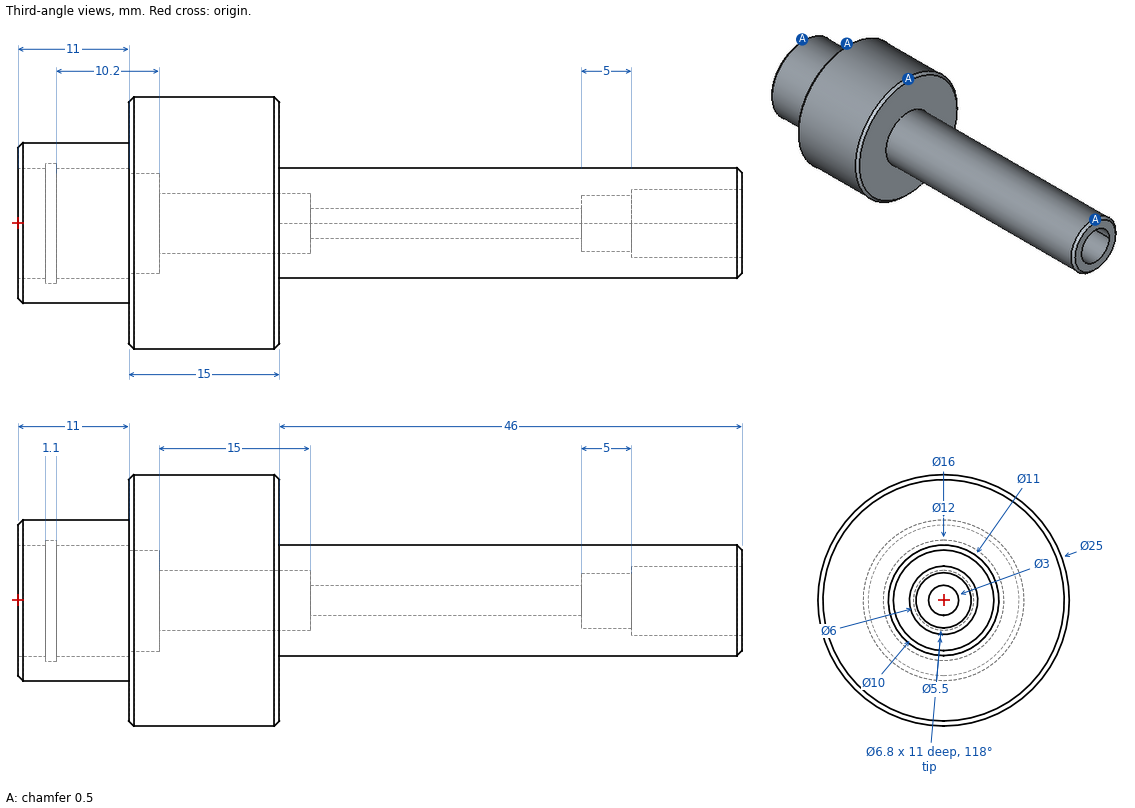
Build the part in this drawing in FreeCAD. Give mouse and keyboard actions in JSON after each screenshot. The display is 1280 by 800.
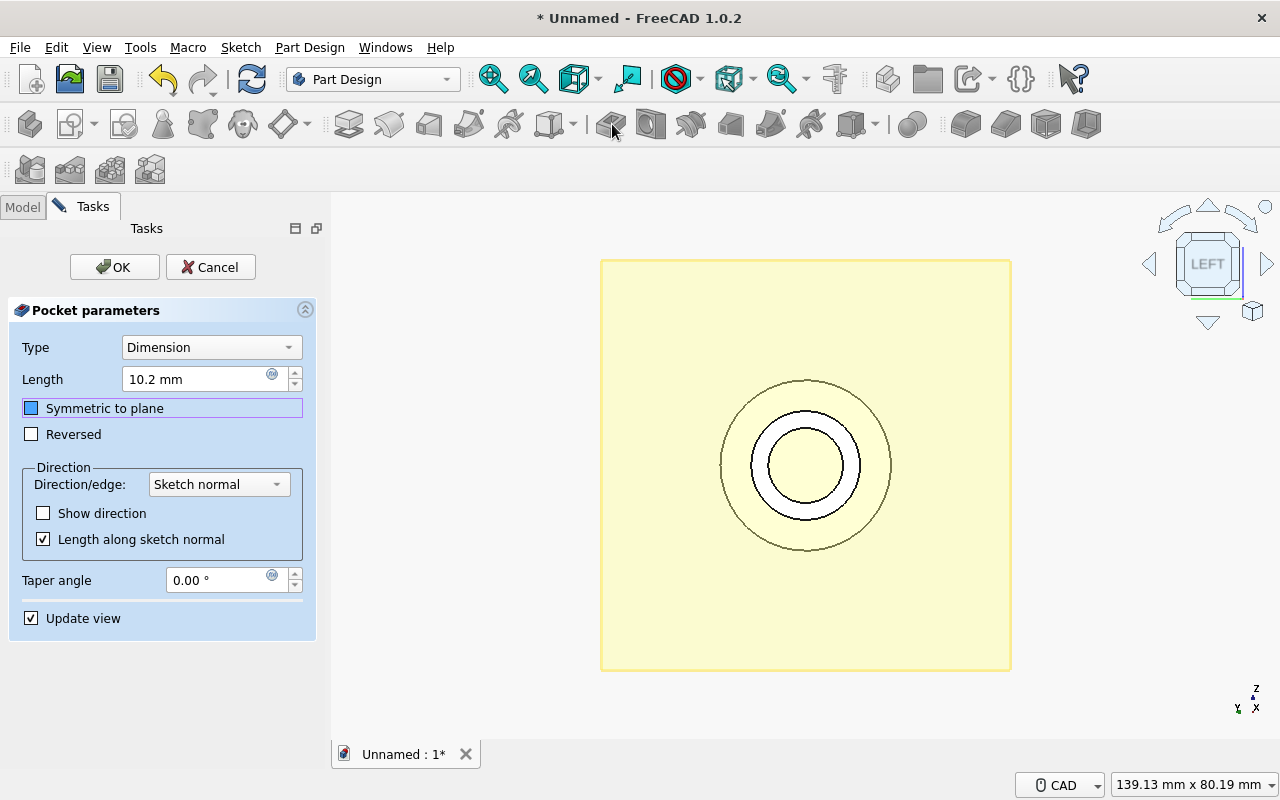
{"action": "left_click", "coordinate": [30, 434]}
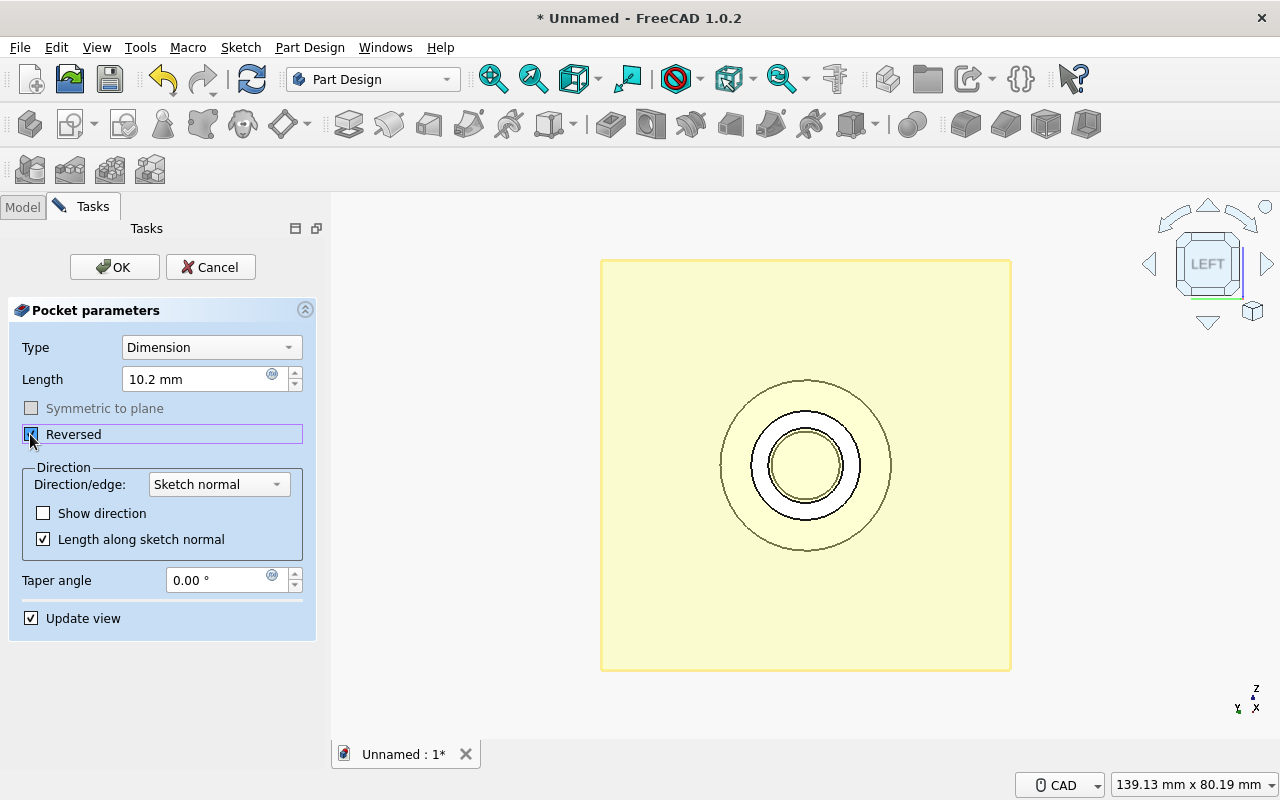
{"action": "left_click", "coordinate": [115, 267]}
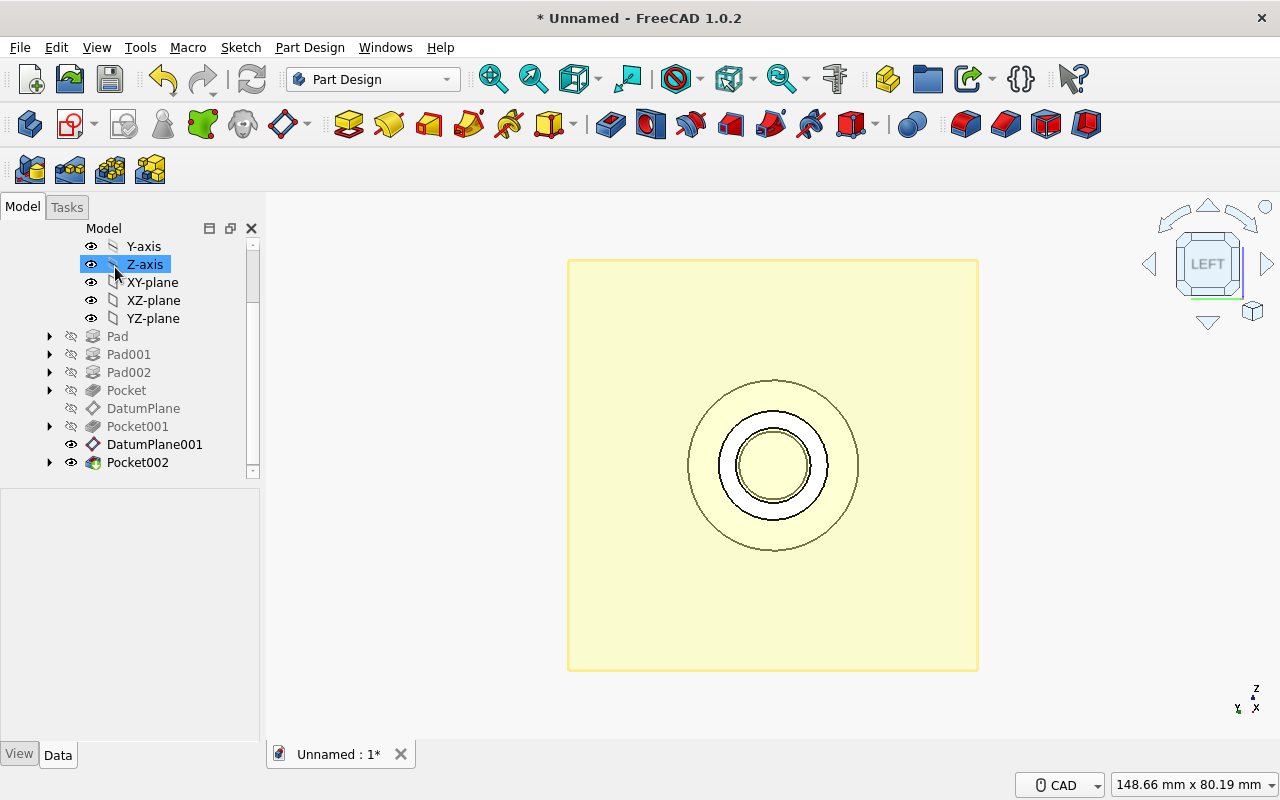
{"action": "left_click", "coordinate": [116, 444]}
{"action": "key", "text": "space"}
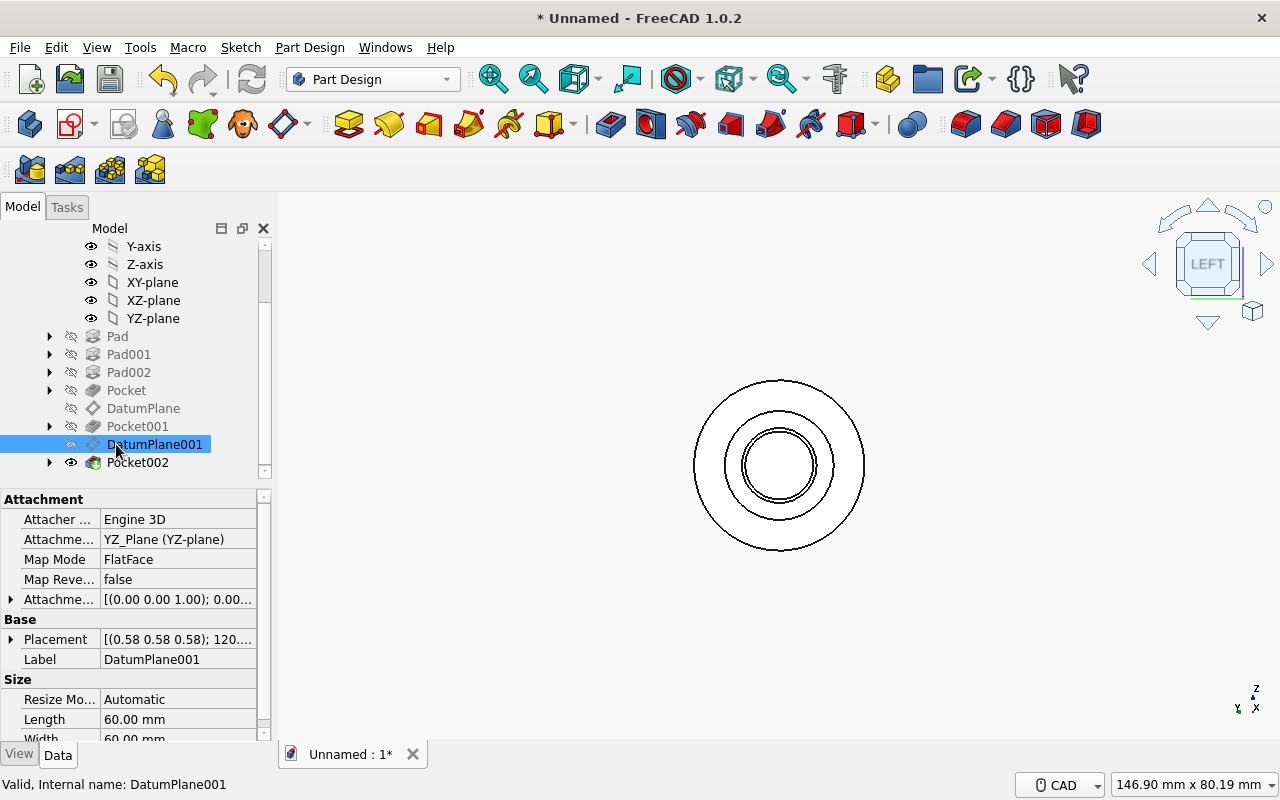
{"action": "left_click", "coordinate": [494, 80]}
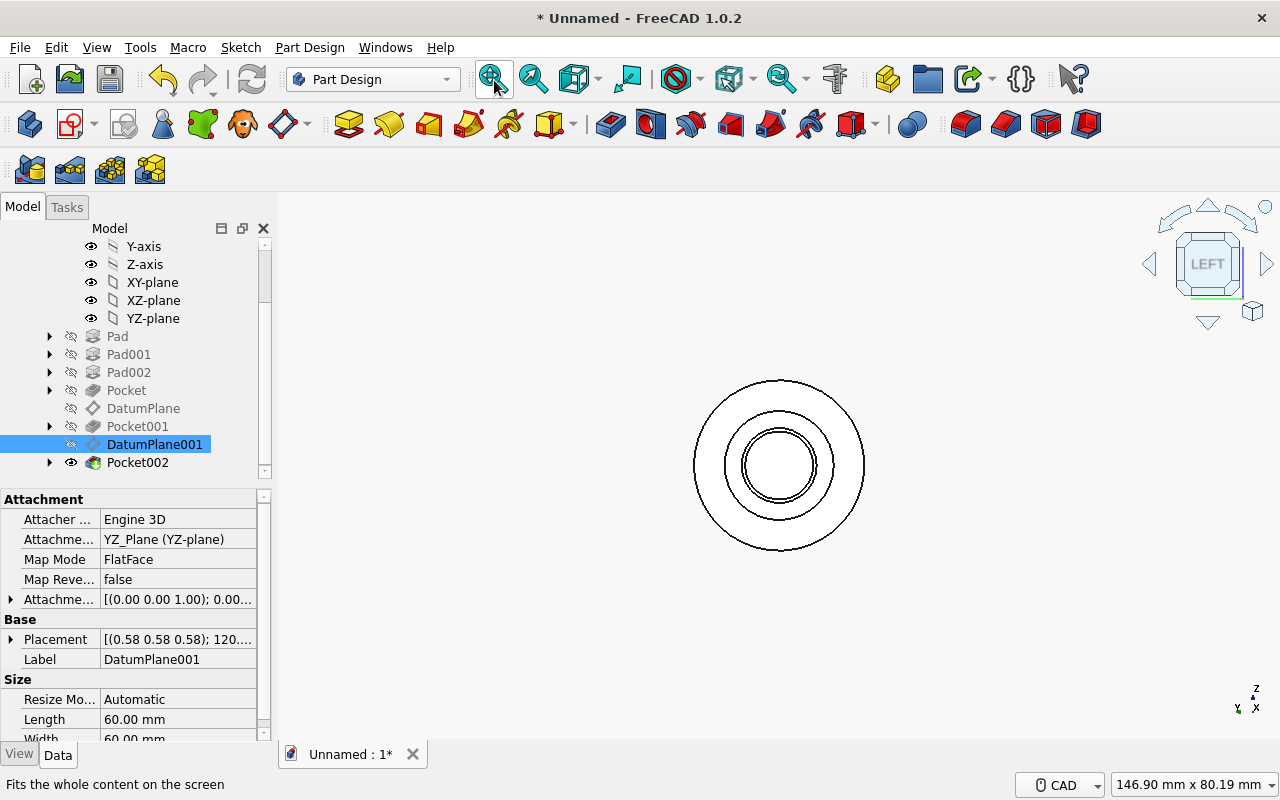
{"action": "left_click", "coordinate": [779, 464]}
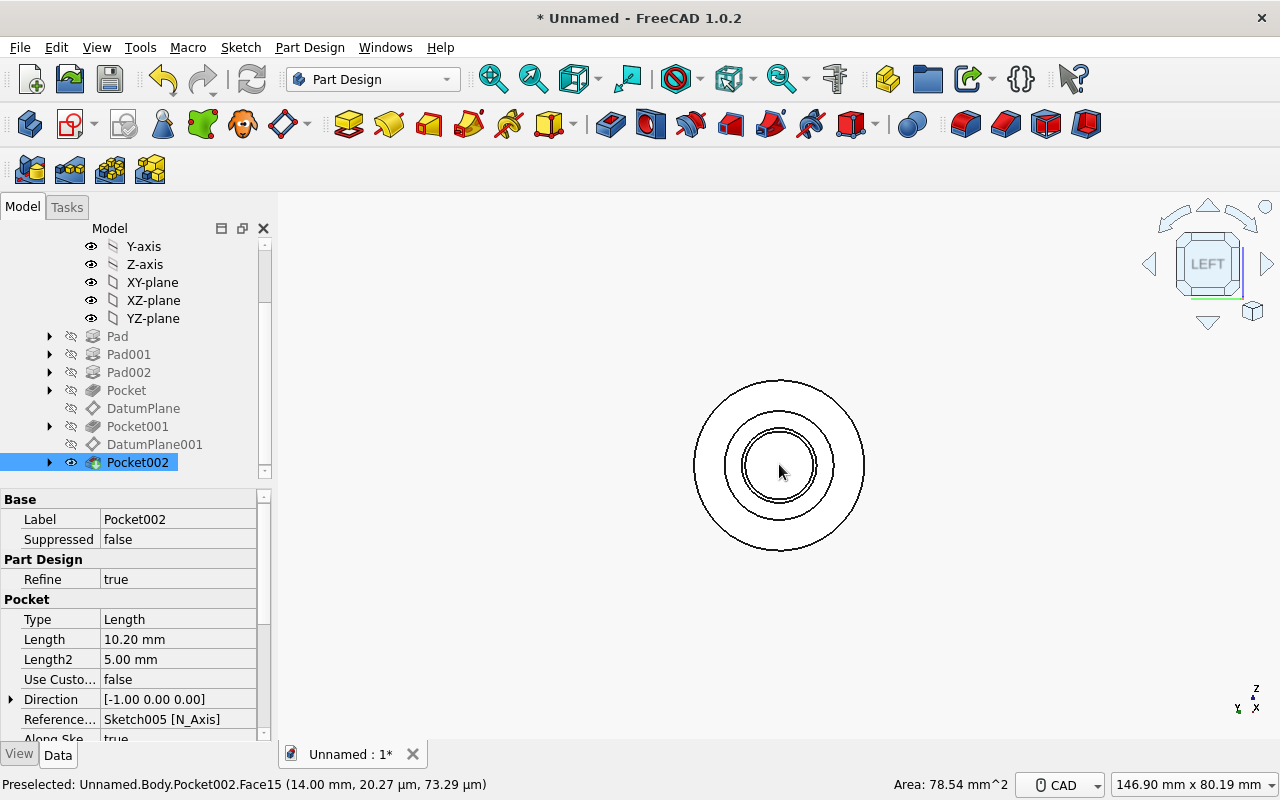
{"action": "left_click", "coordinate": [70, 124]}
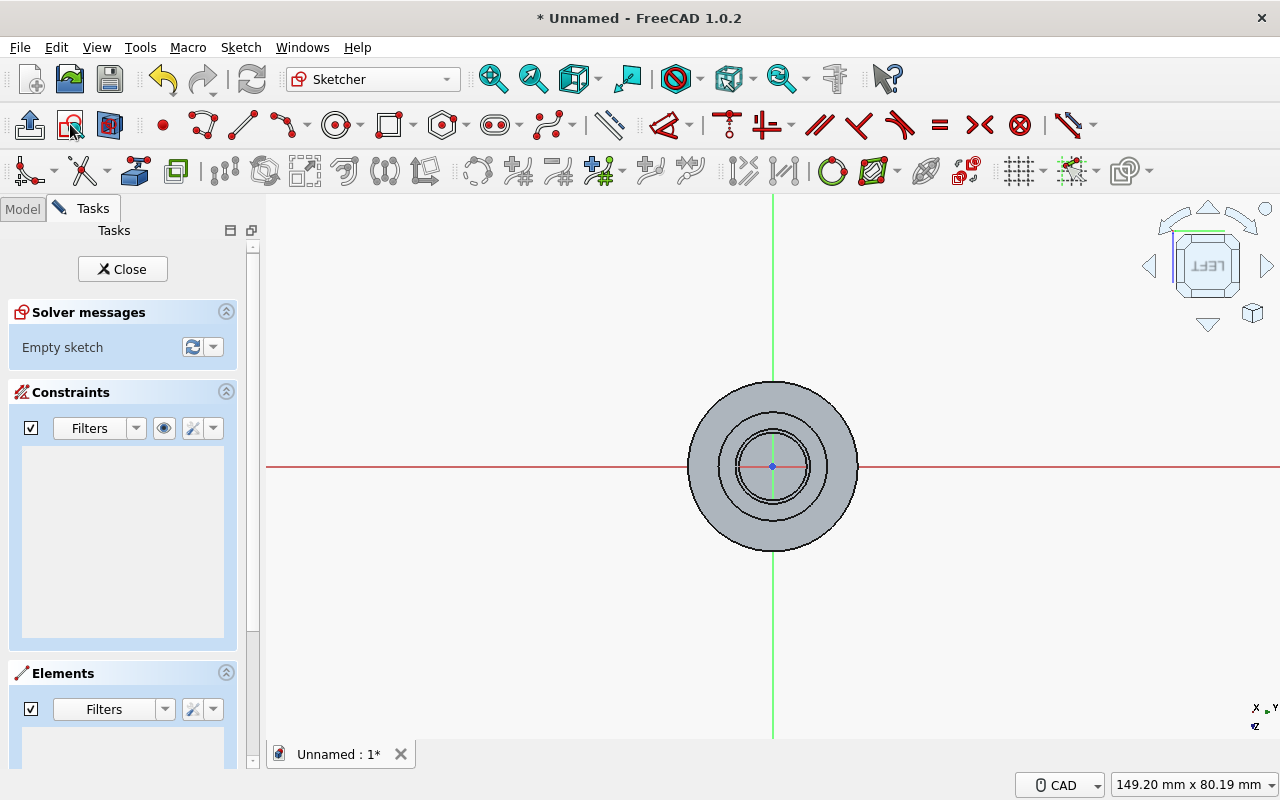
{"action": "left_click", "coordinate": [110, 126]}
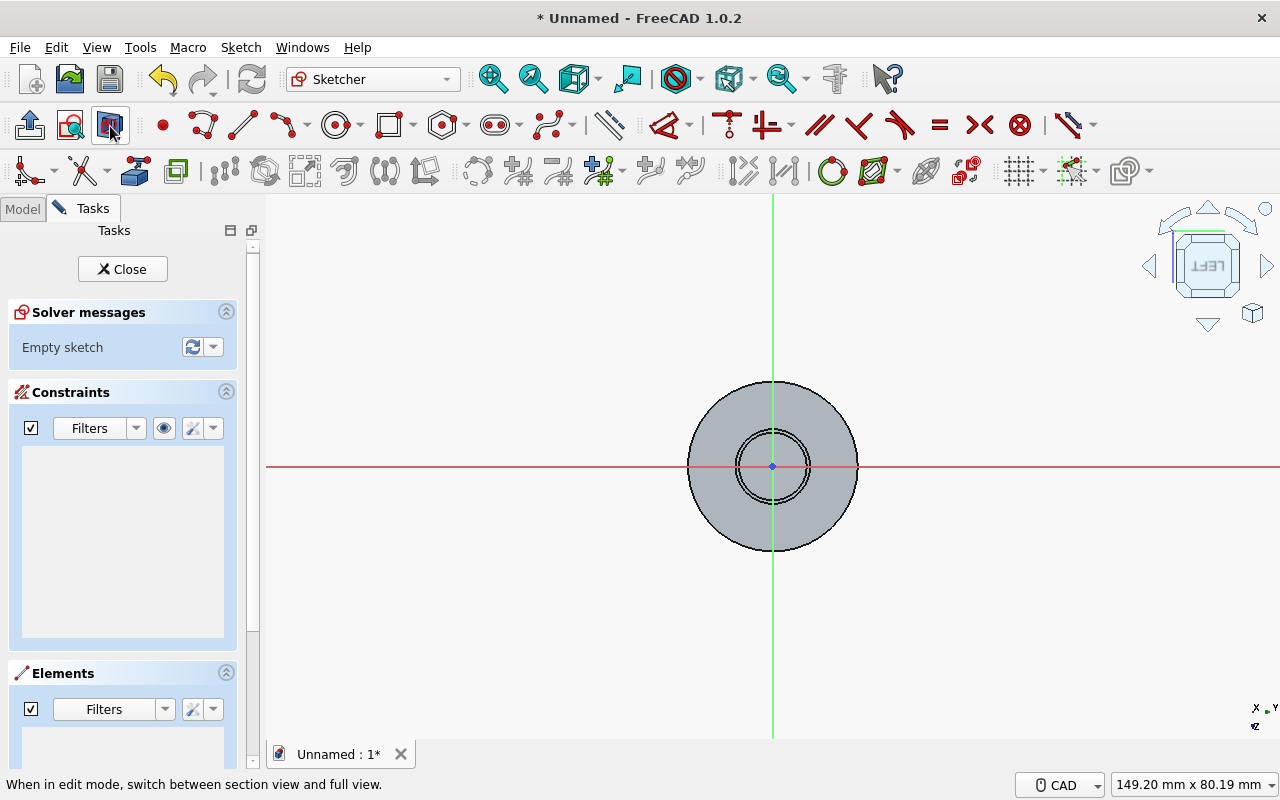
{"action": "scroll", "coordinate": [781, 466], "scroll_direction": "up", "scroll_amount": 11}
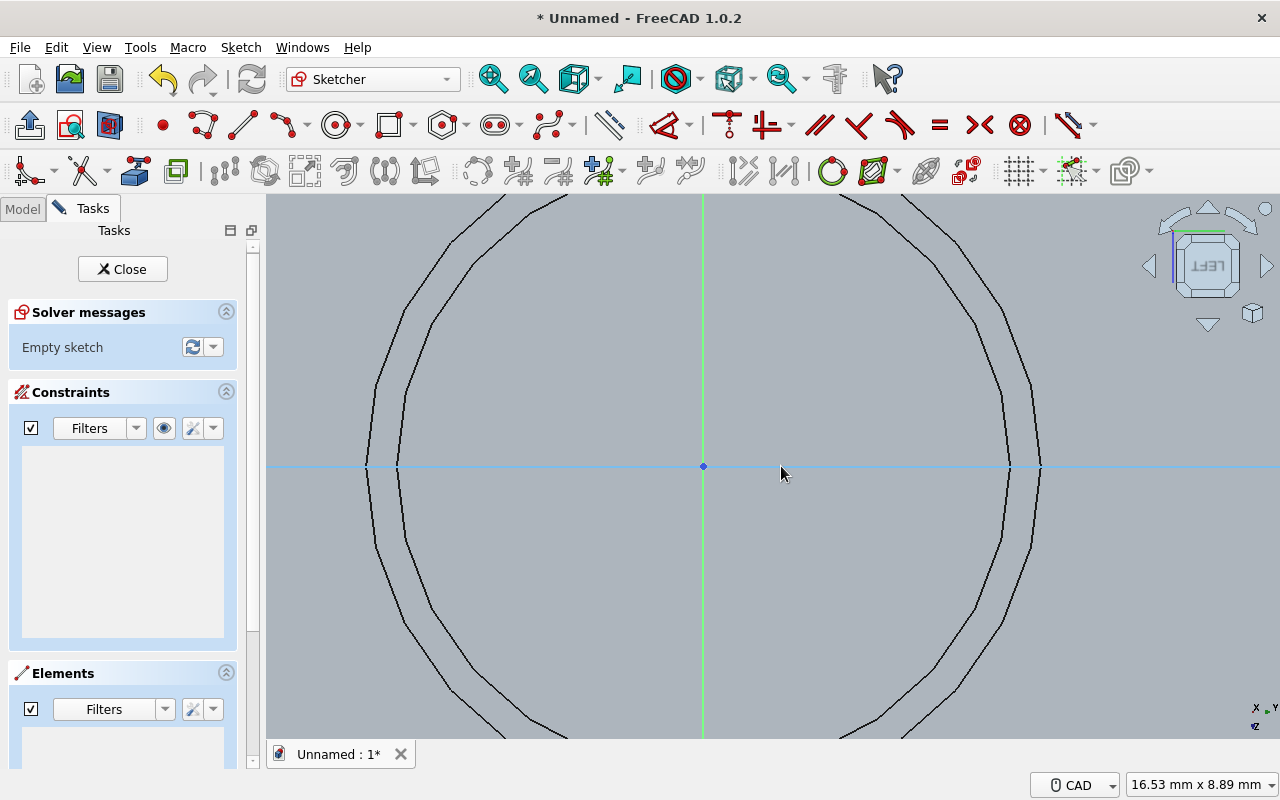
{"action": "left_click", "coordinate": [336, 126]}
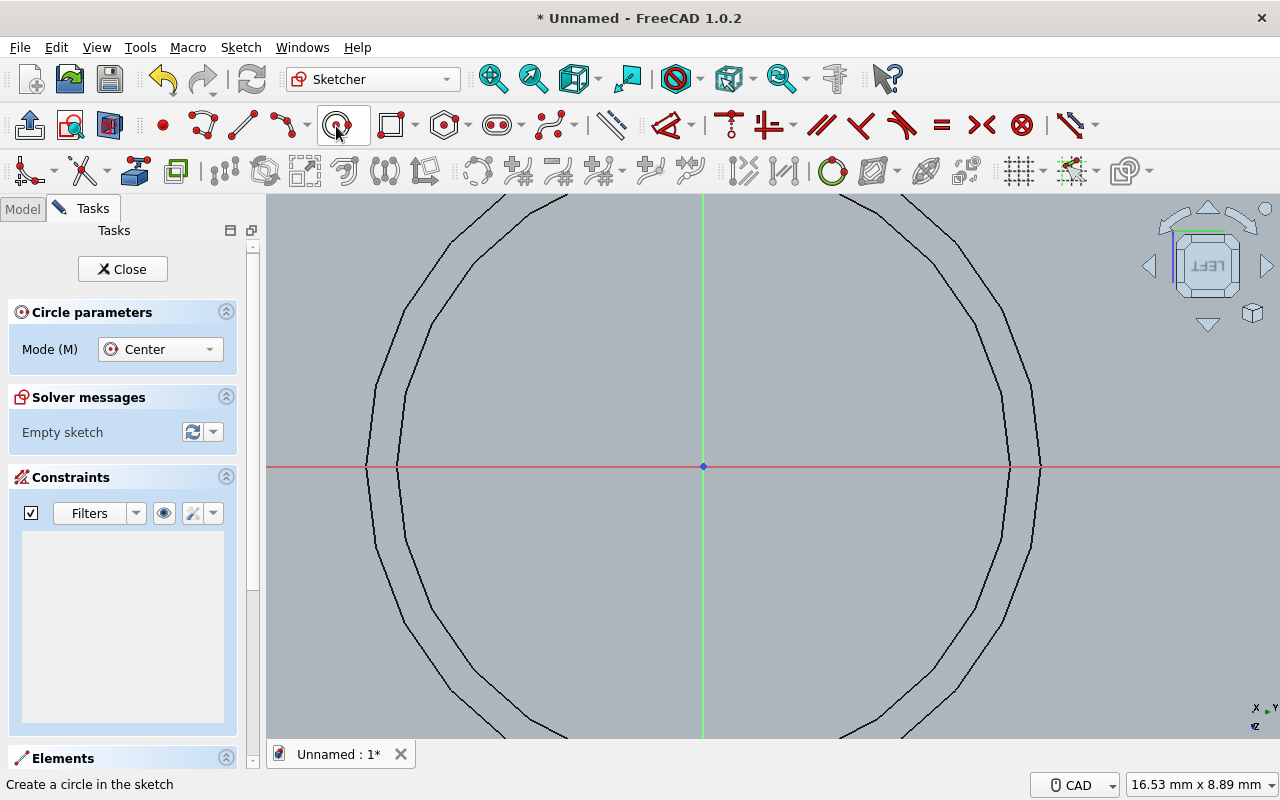
{"action": "left_click", "coordinate": [703, 467]}
{"action": "mouse_move", "coordinate": [834, 336]}